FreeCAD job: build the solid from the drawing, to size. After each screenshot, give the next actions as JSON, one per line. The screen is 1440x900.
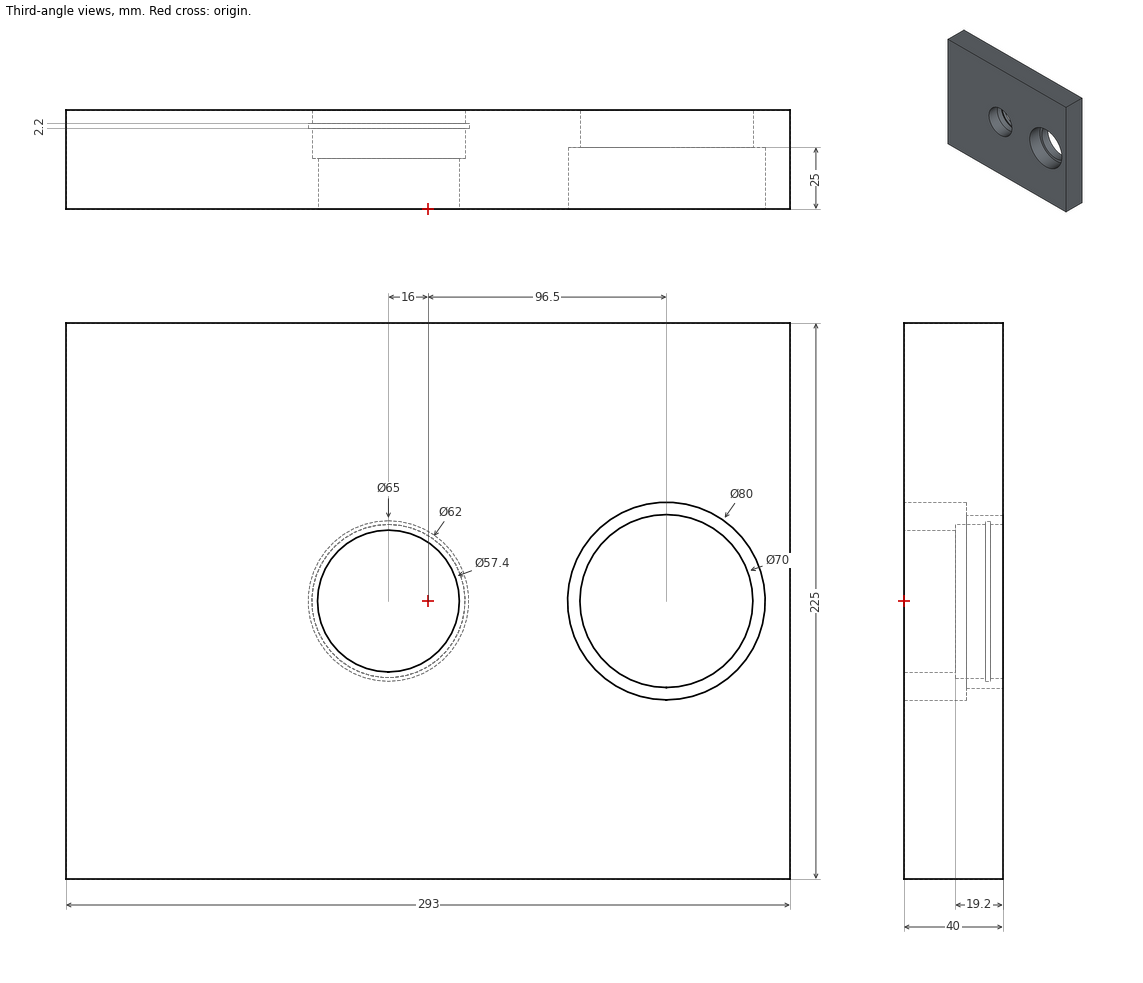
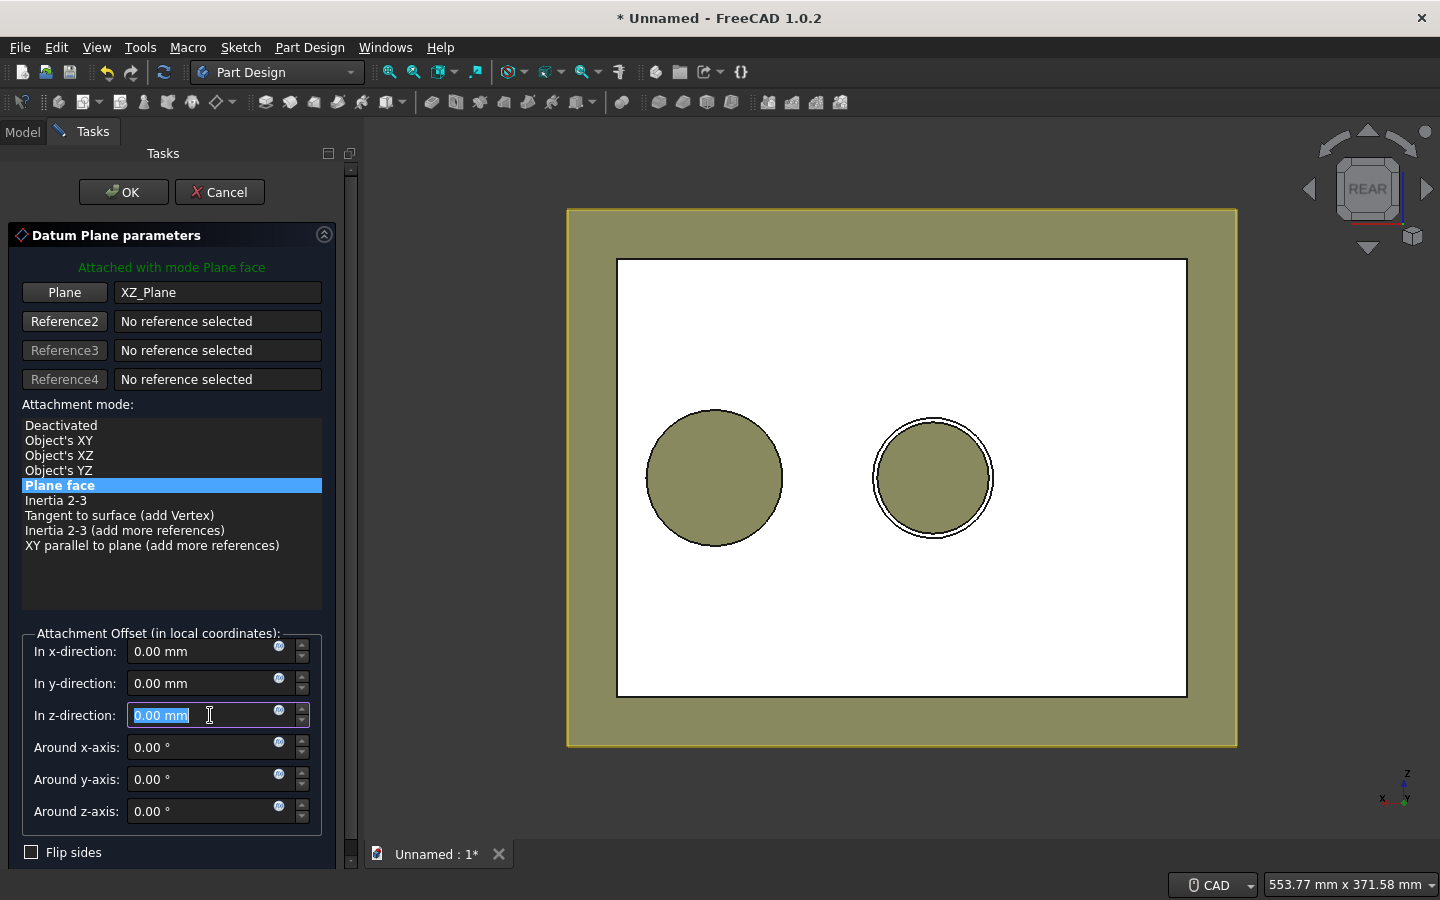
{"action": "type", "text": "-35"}
{"action": "key", "text": "Tab"}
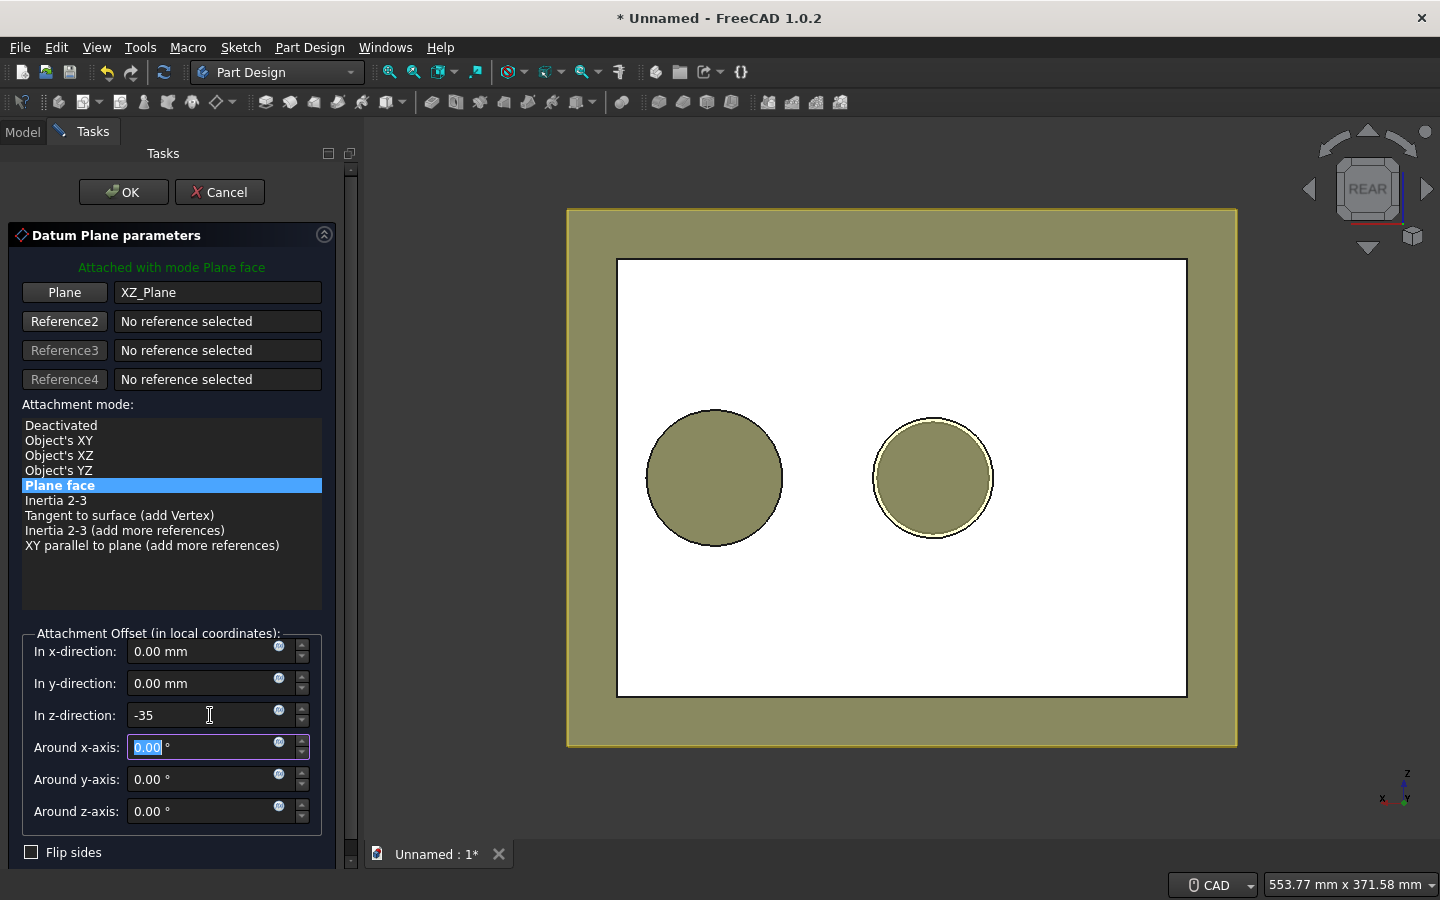
{"action": "left_click", "coordinate": [124, 192]}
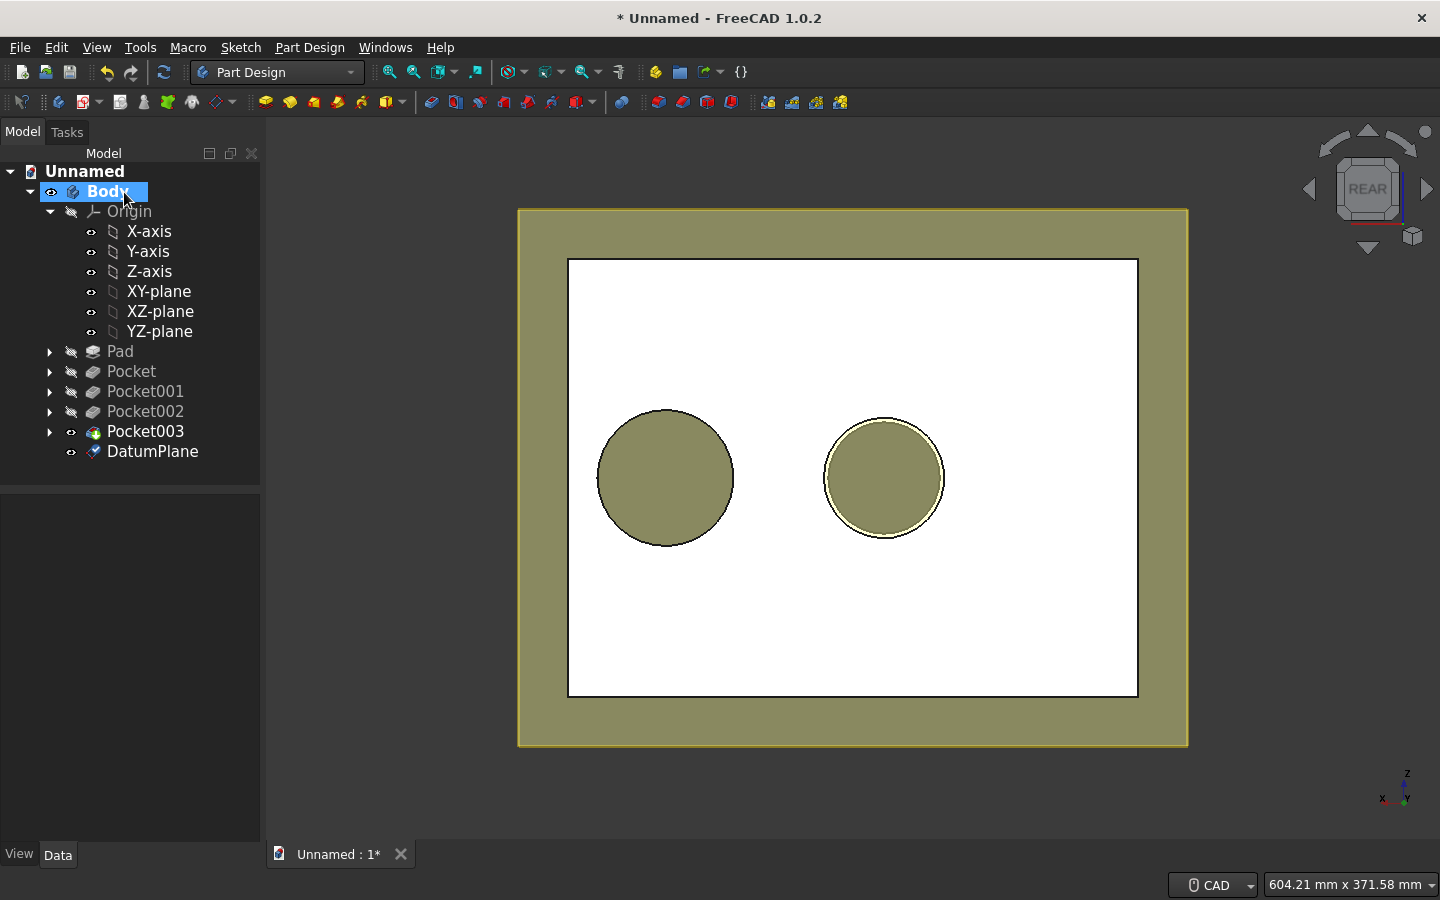
{"action": "left_click", "coordinate": [116, 452]}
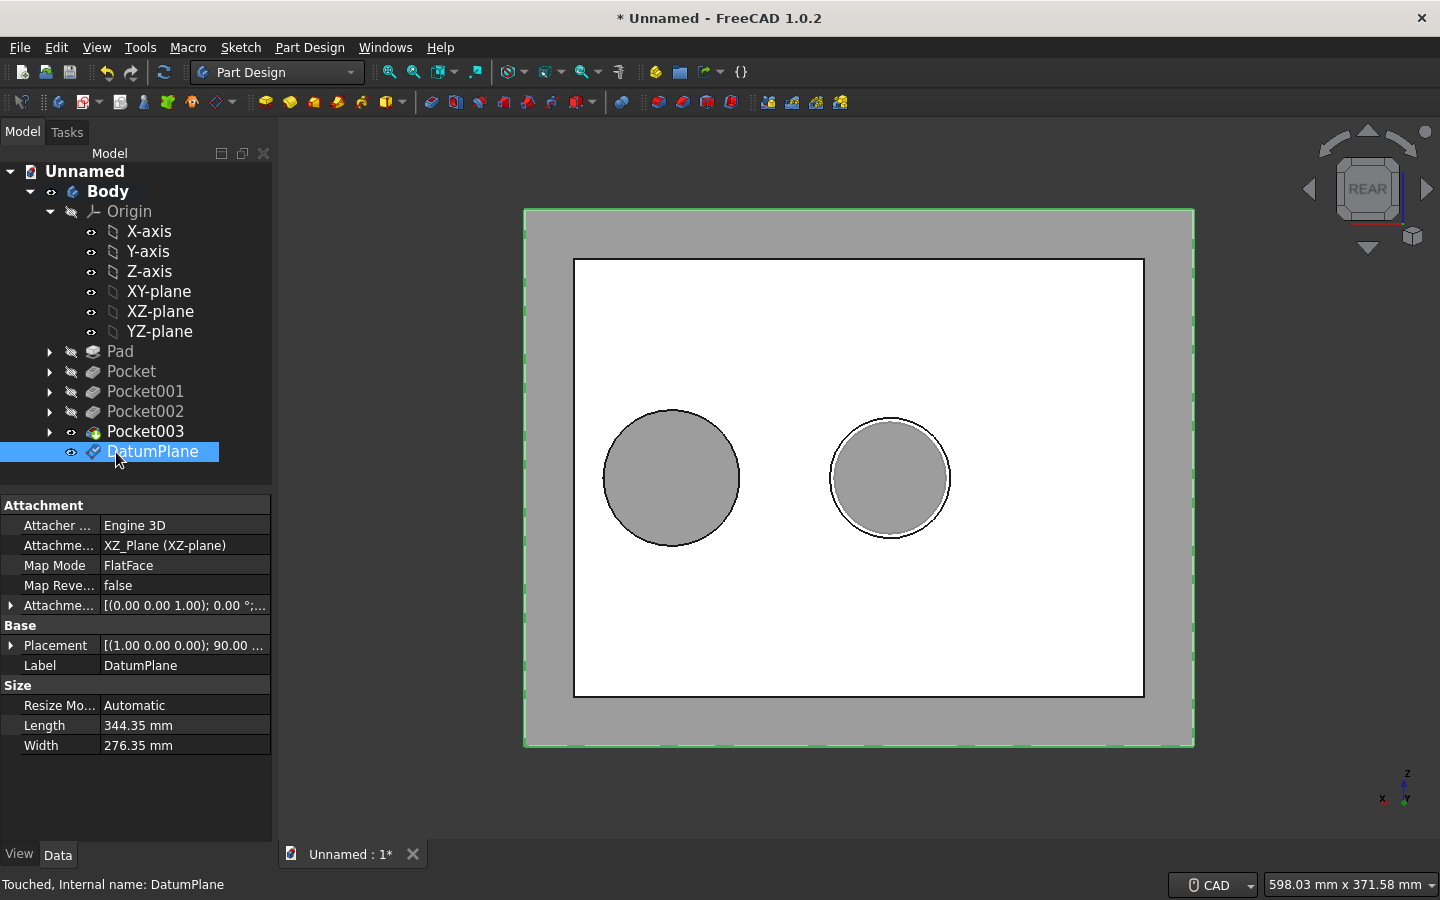
{"action": "left_click", "coordinate": [84, 102]}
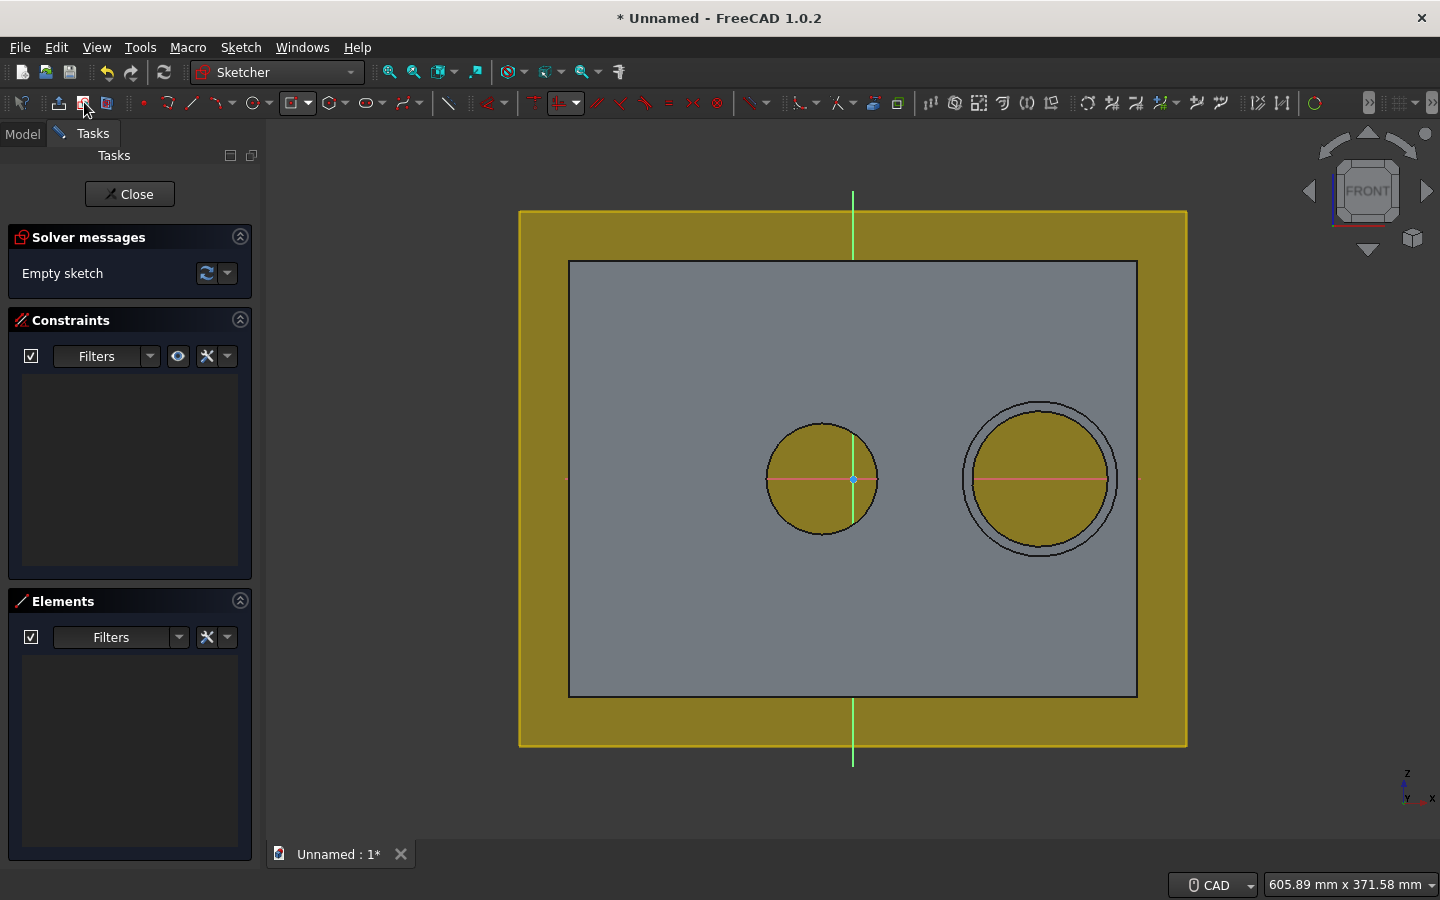
{"action": "left_click", "coordinate": [108, 104]}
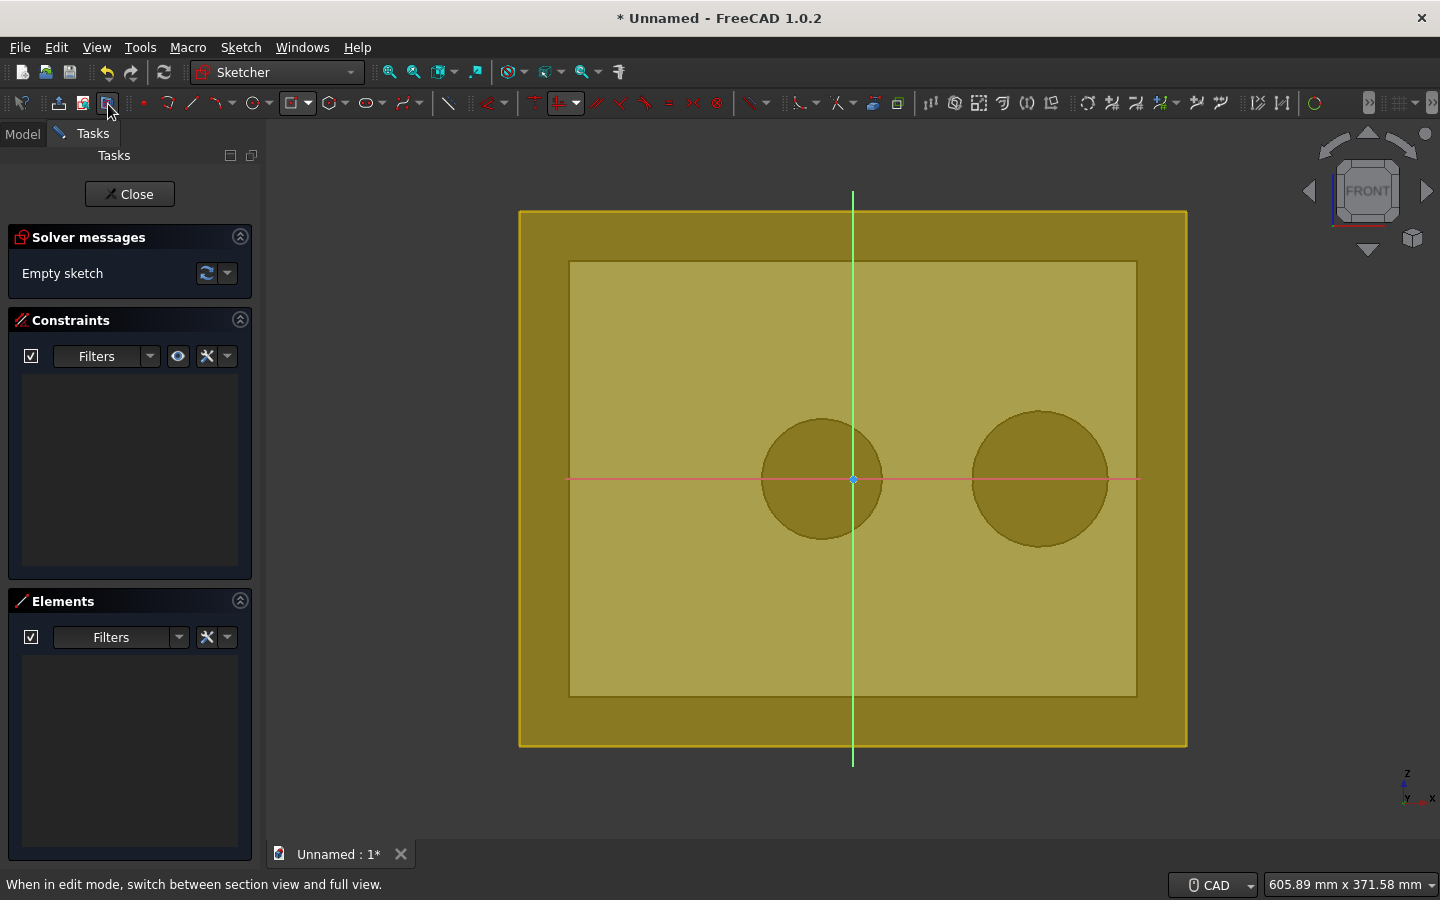
{"action": "scroll", "coordinate": [834, 479], "scroll_direction": "up", "scroll_amount": 7}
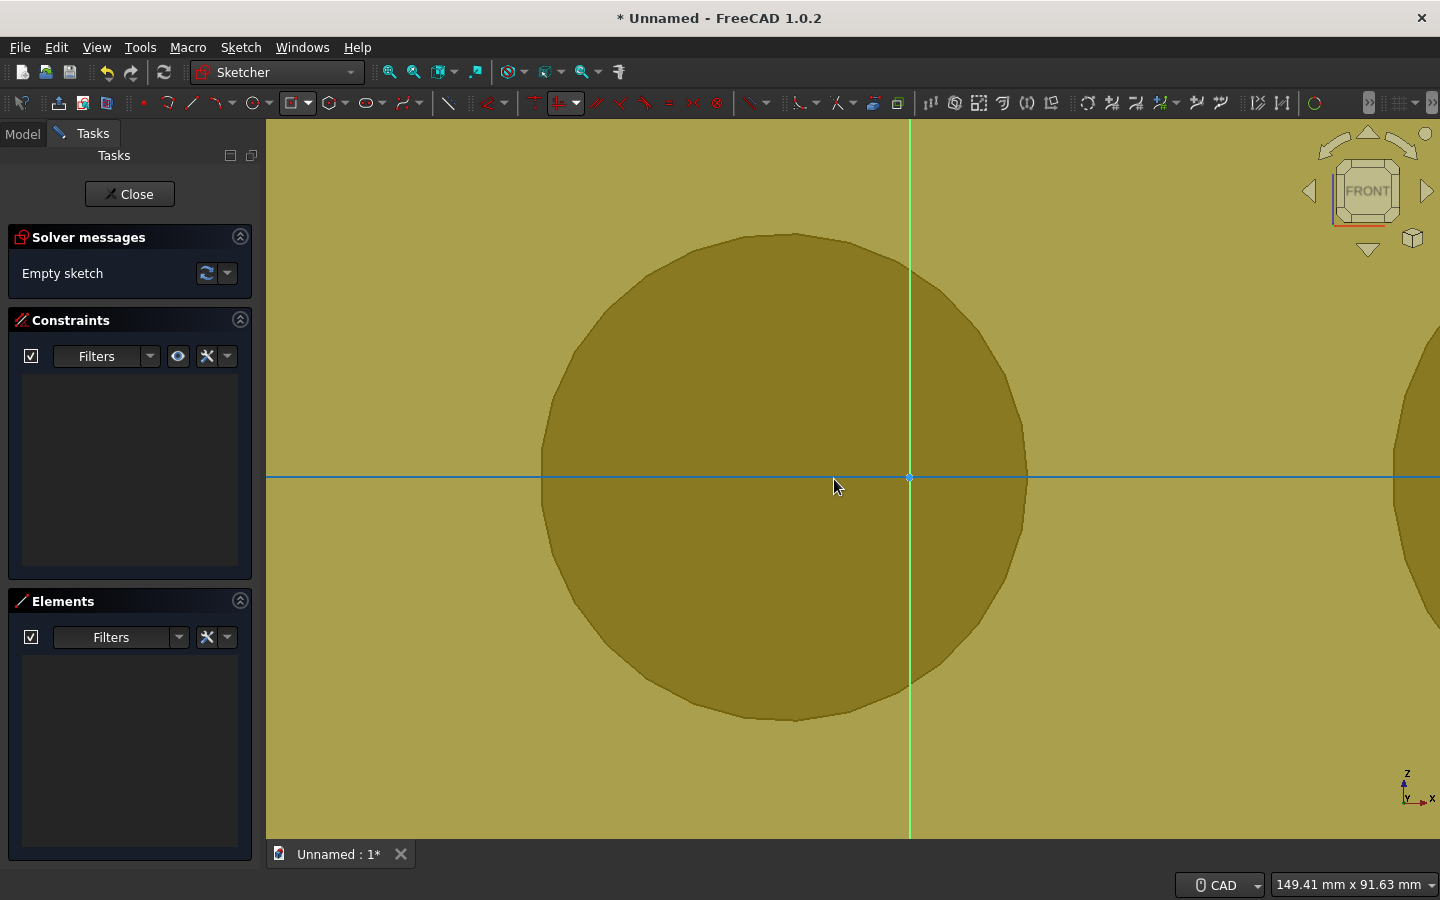
{"action": "left_click", "coordinate": [254, 104]}